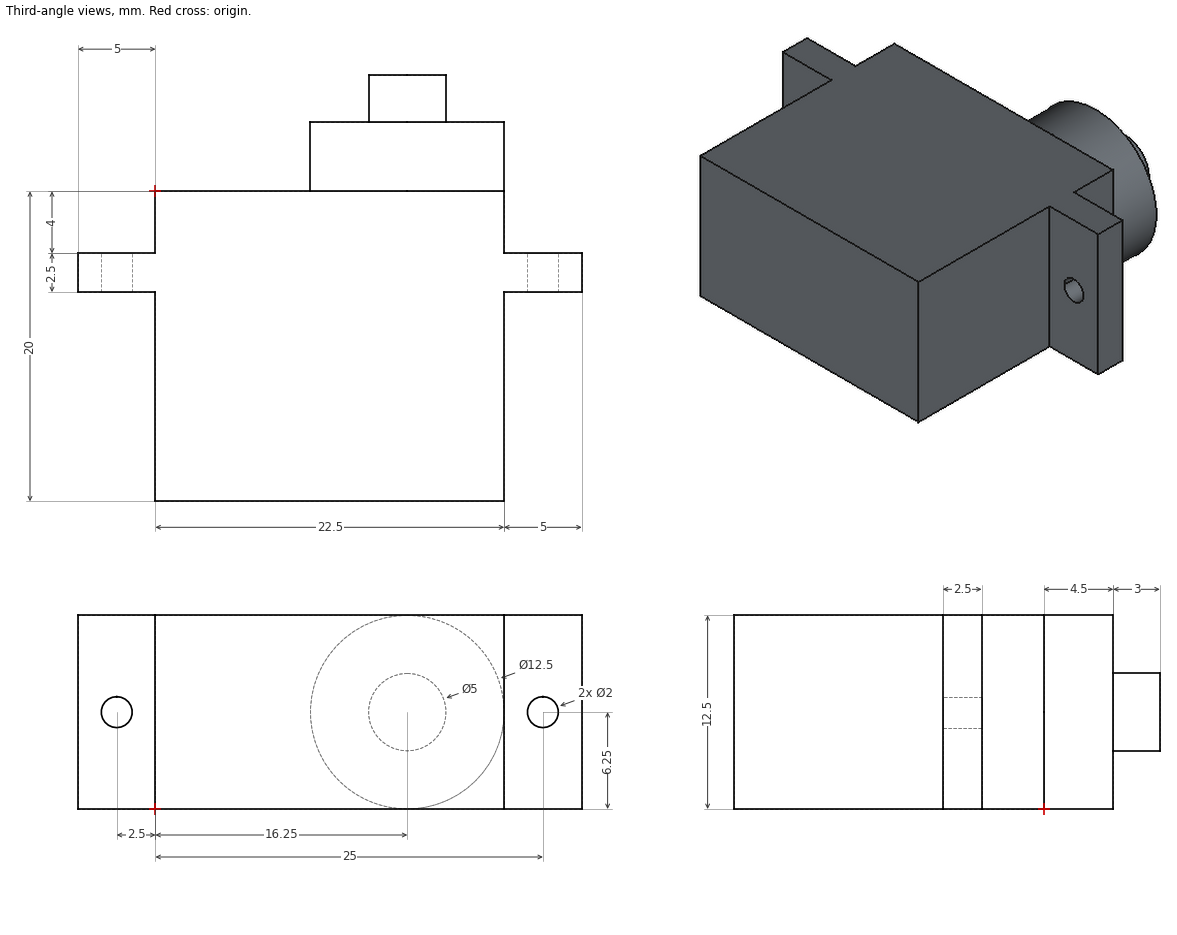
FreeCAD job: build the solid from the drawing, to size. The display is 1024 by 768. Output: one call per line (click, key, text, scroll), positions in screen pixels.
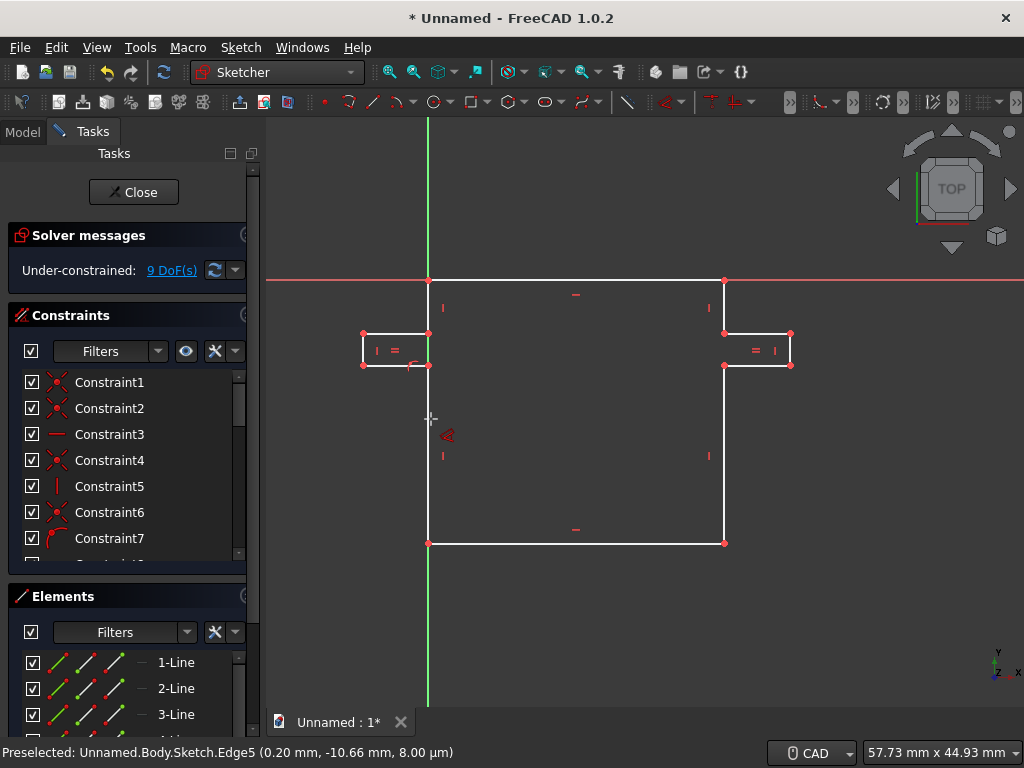
click(428, 296)
click(394, 307)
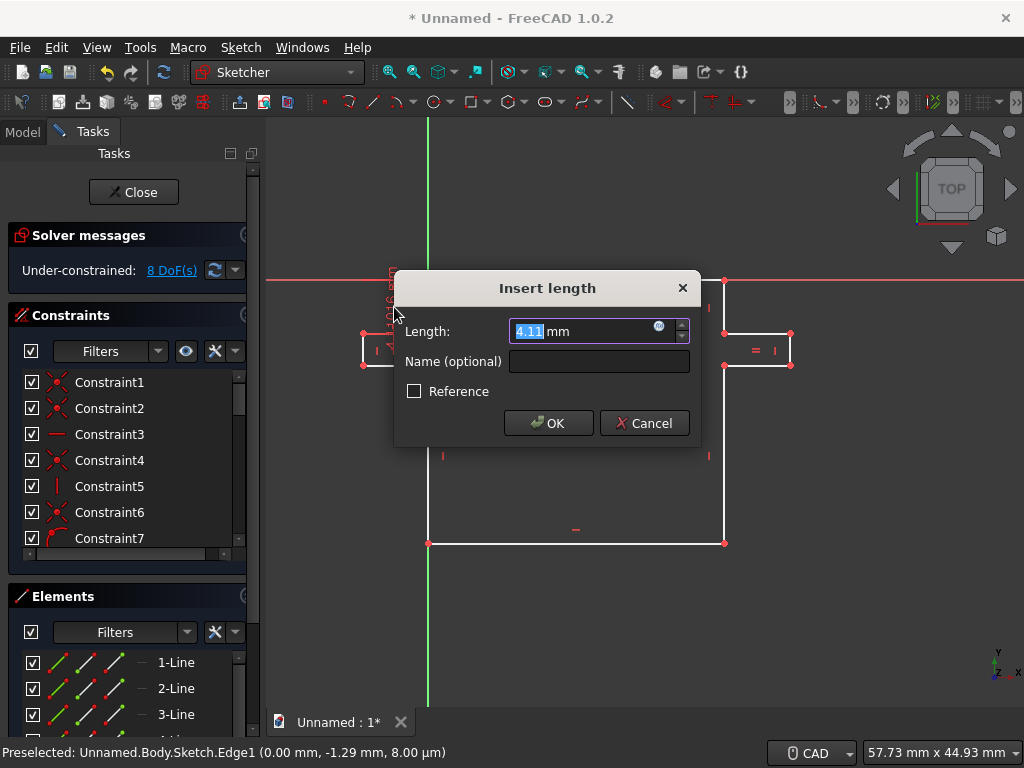
text(4)
key(Return)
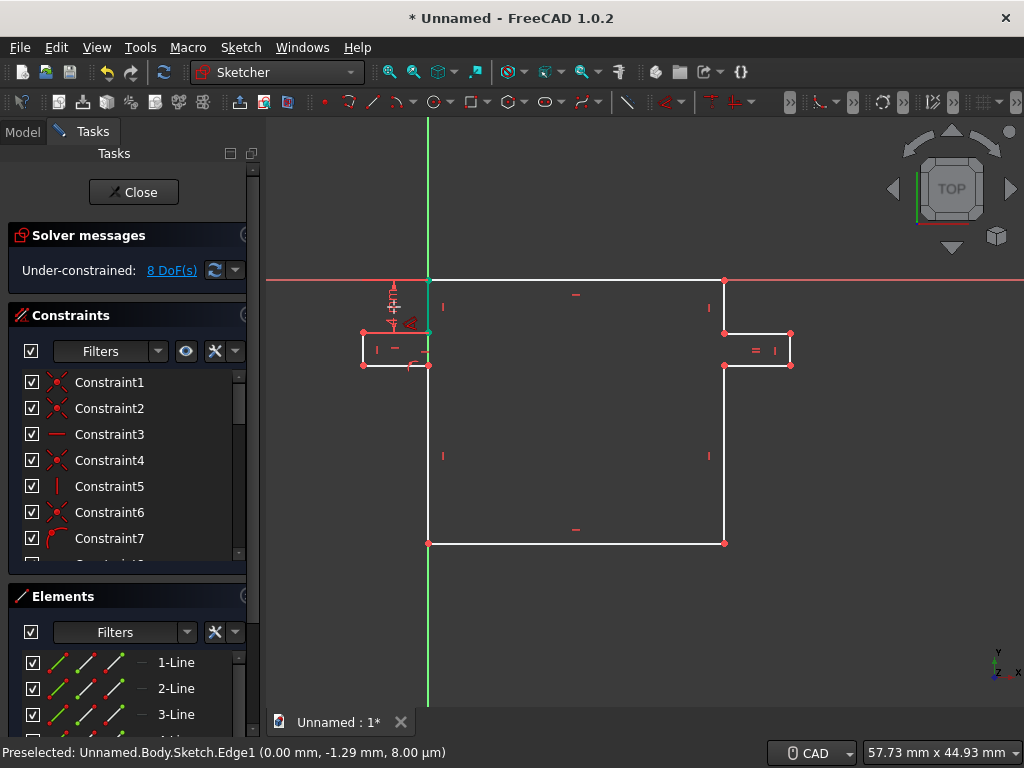
click(409, 333)
click(396, 391)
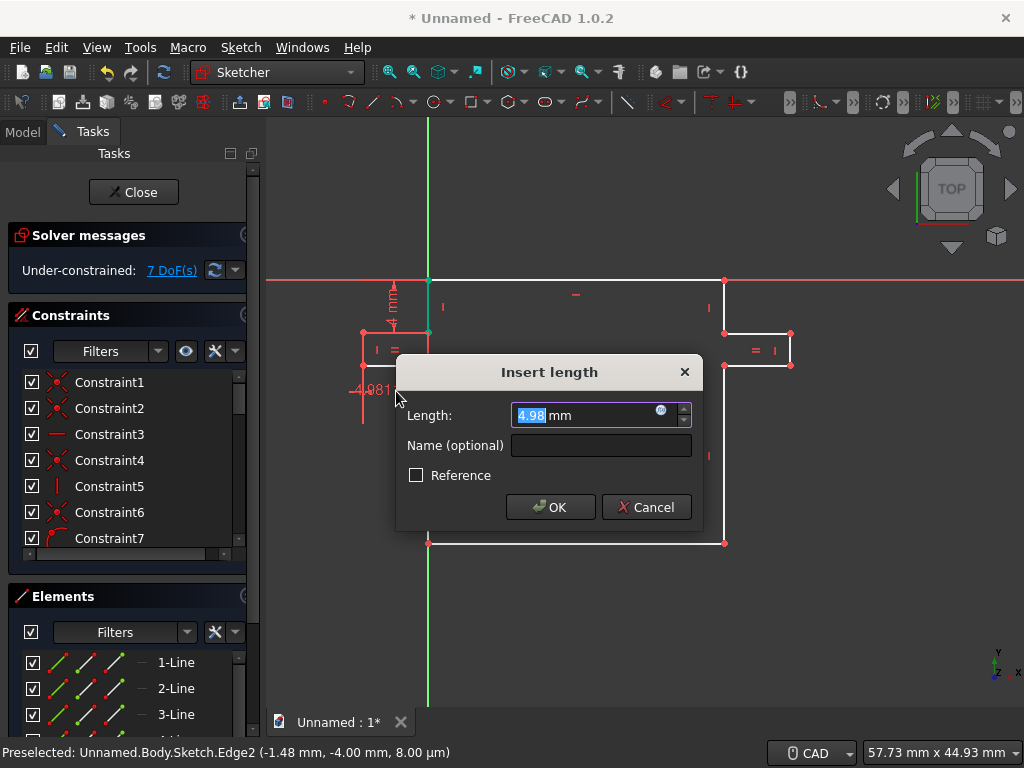
text(5)
key(Return)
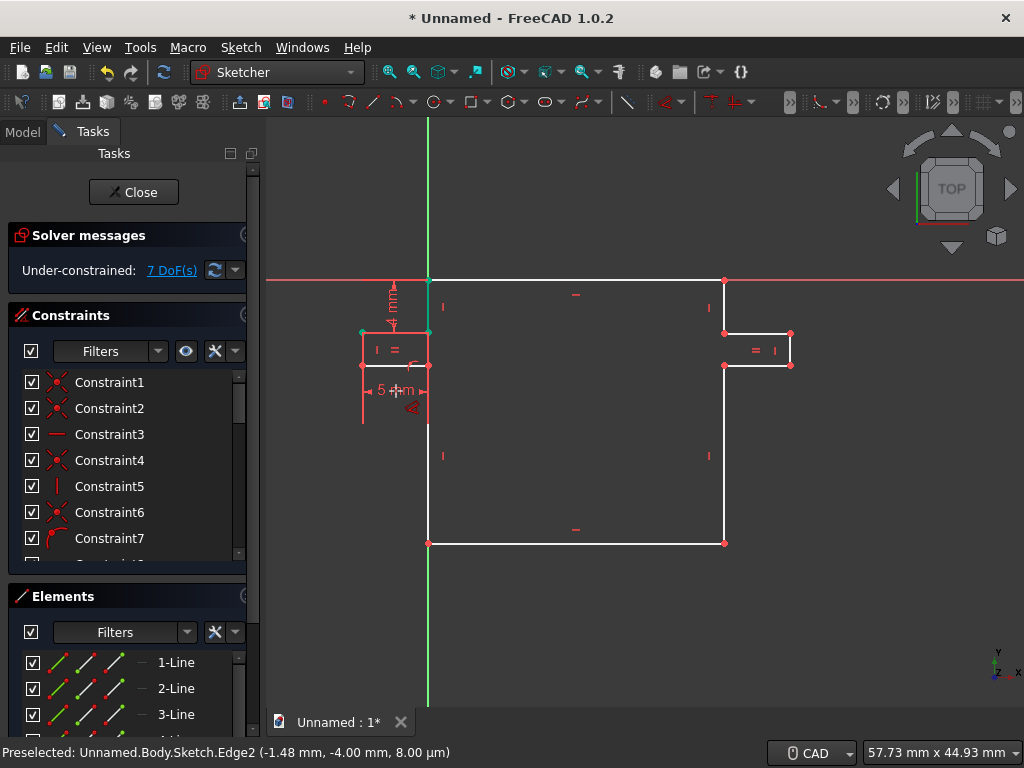
click(744, 366)
click(757, 400)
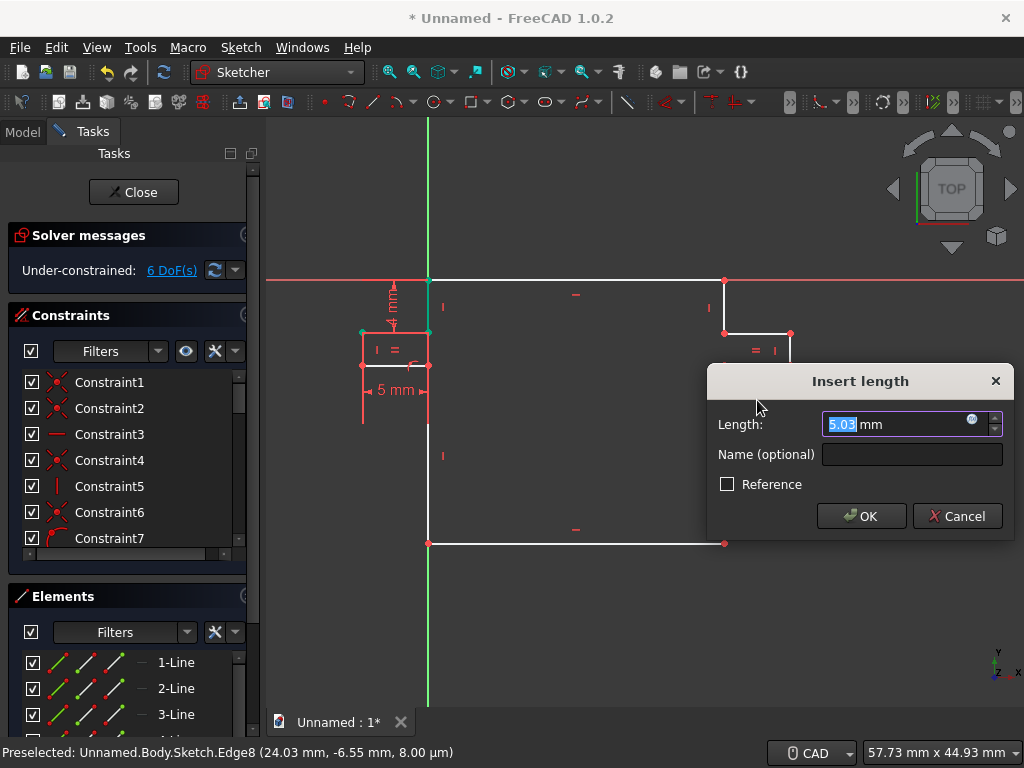
text(5)
key(Return)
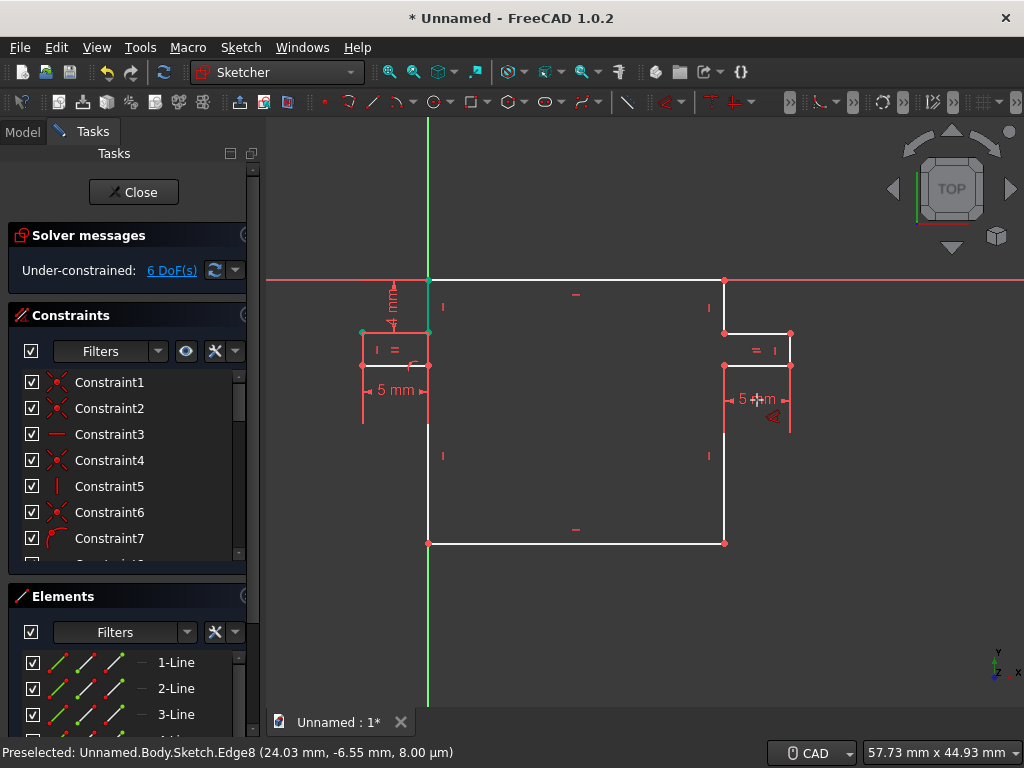
click(770, 334)
click(757, 300)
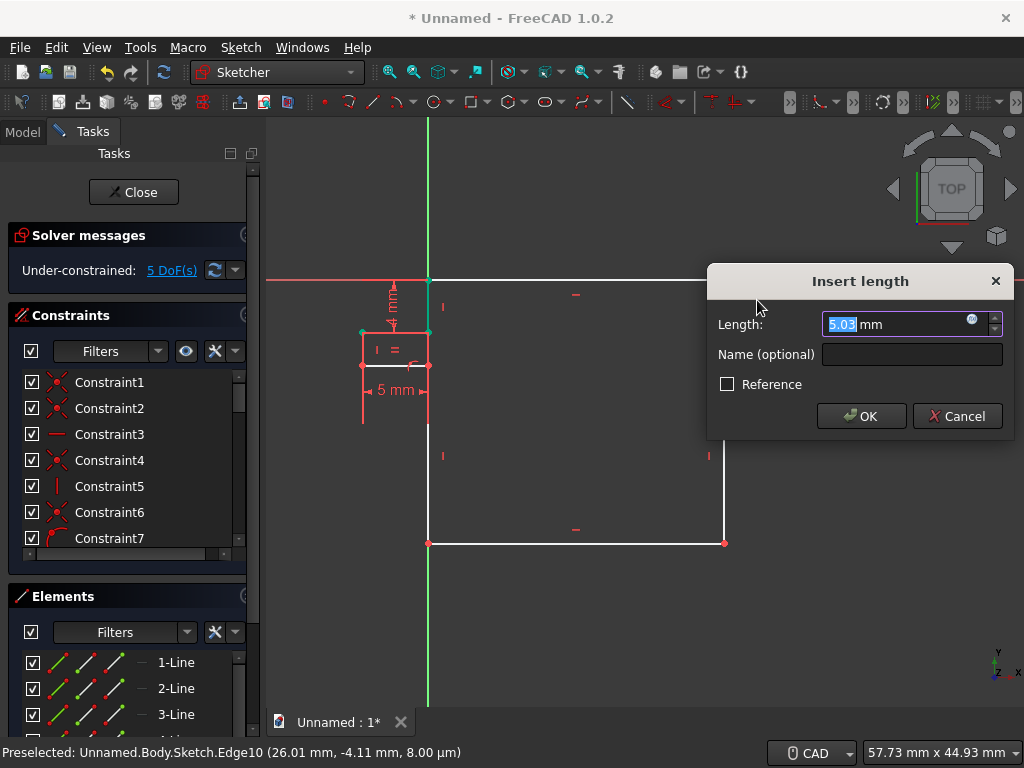
text(5)
key(Return)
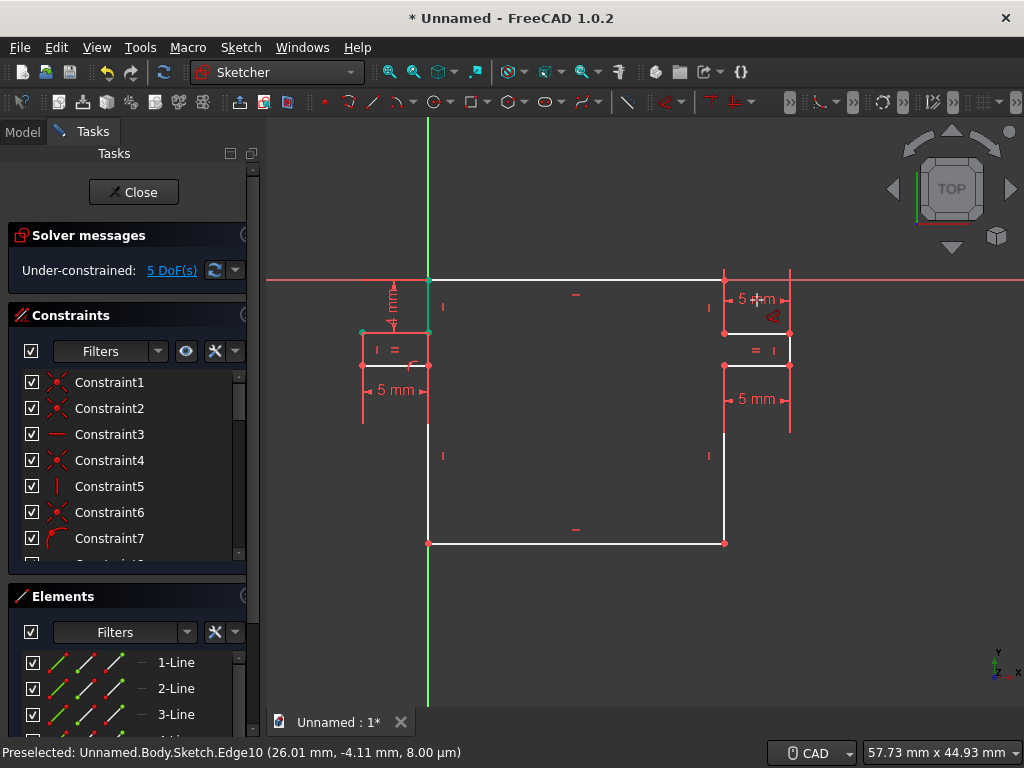
click(724, 318)
click(690, 326)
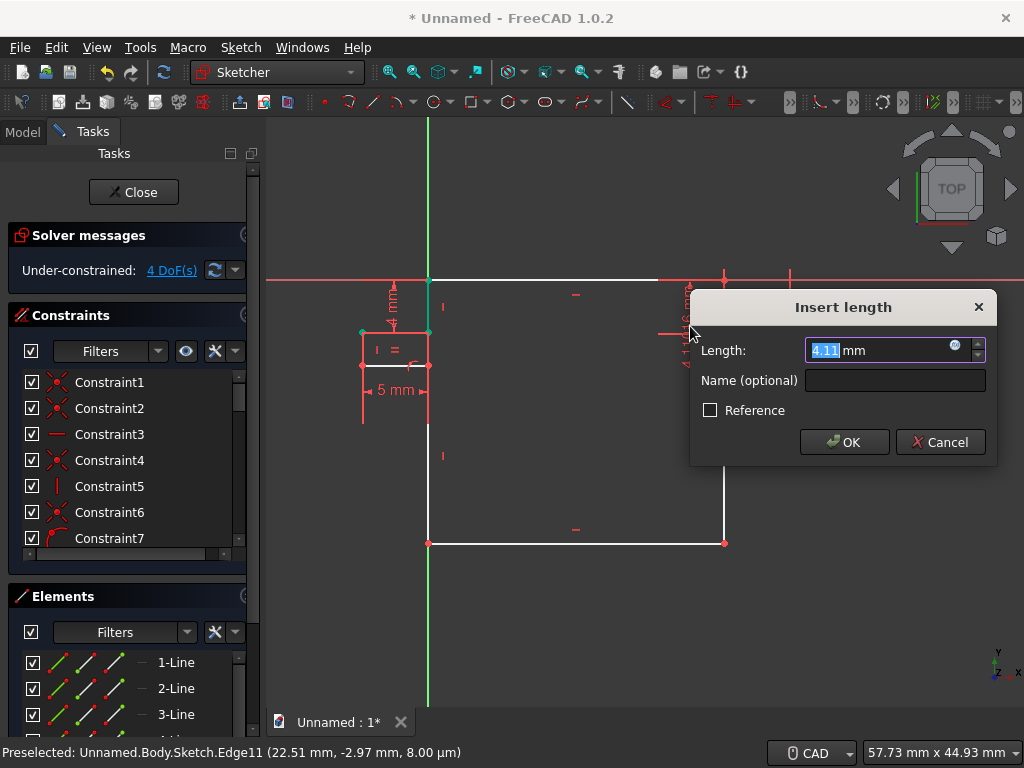
text(4)
key(Return)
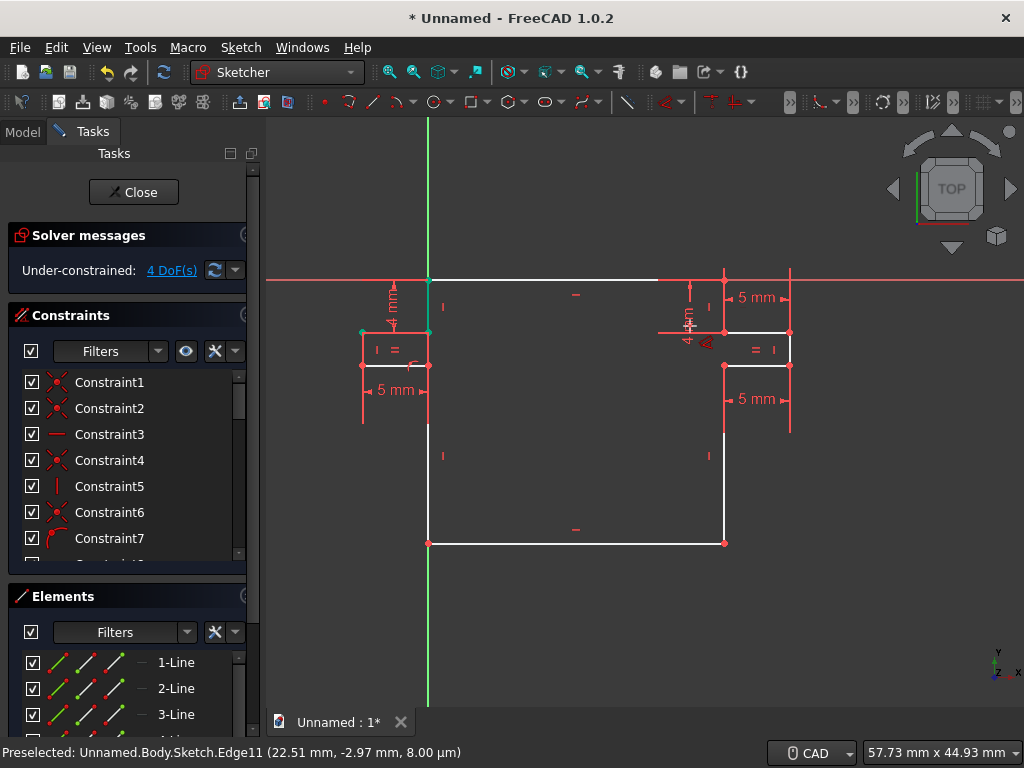
scroll(363, 343, up, 2)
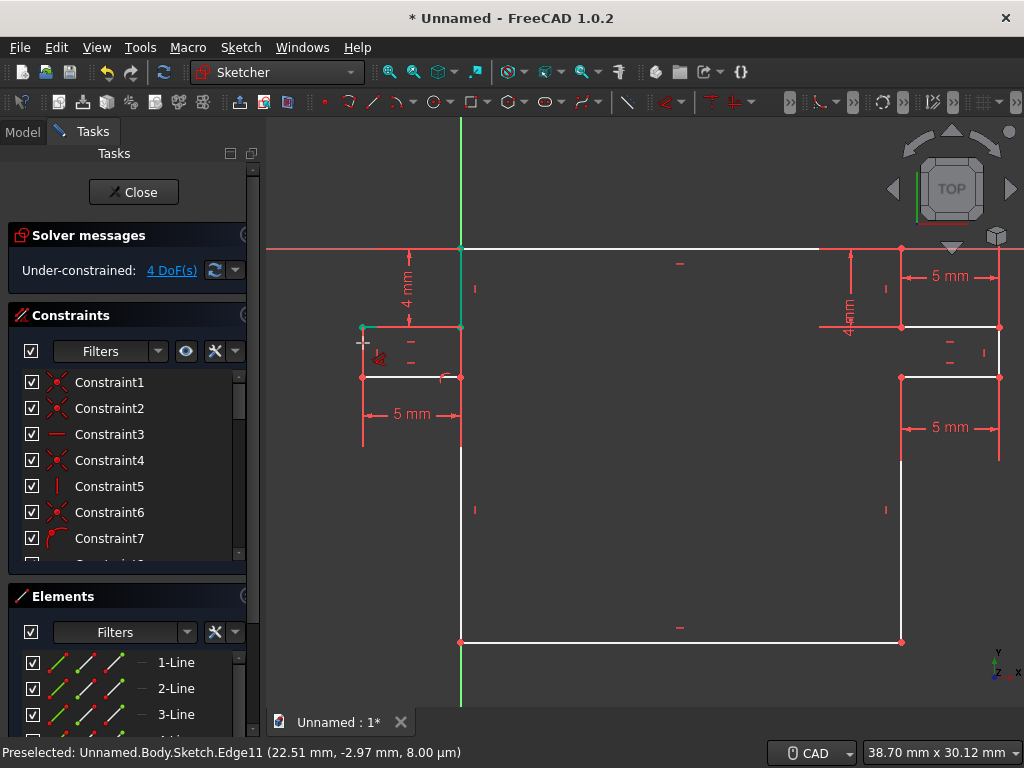
click(363, 342)
click(329, 352)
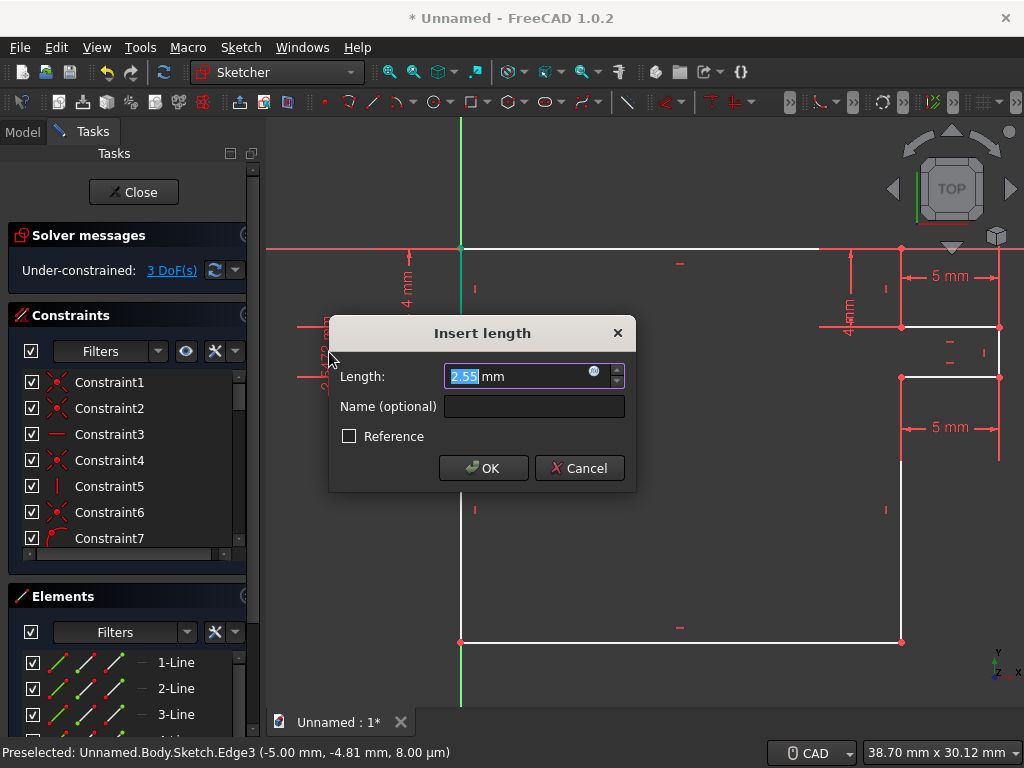
text(2.5)
key(Return)